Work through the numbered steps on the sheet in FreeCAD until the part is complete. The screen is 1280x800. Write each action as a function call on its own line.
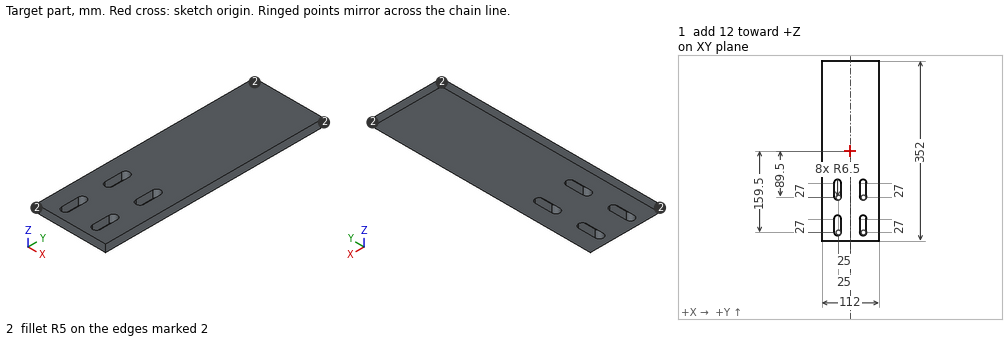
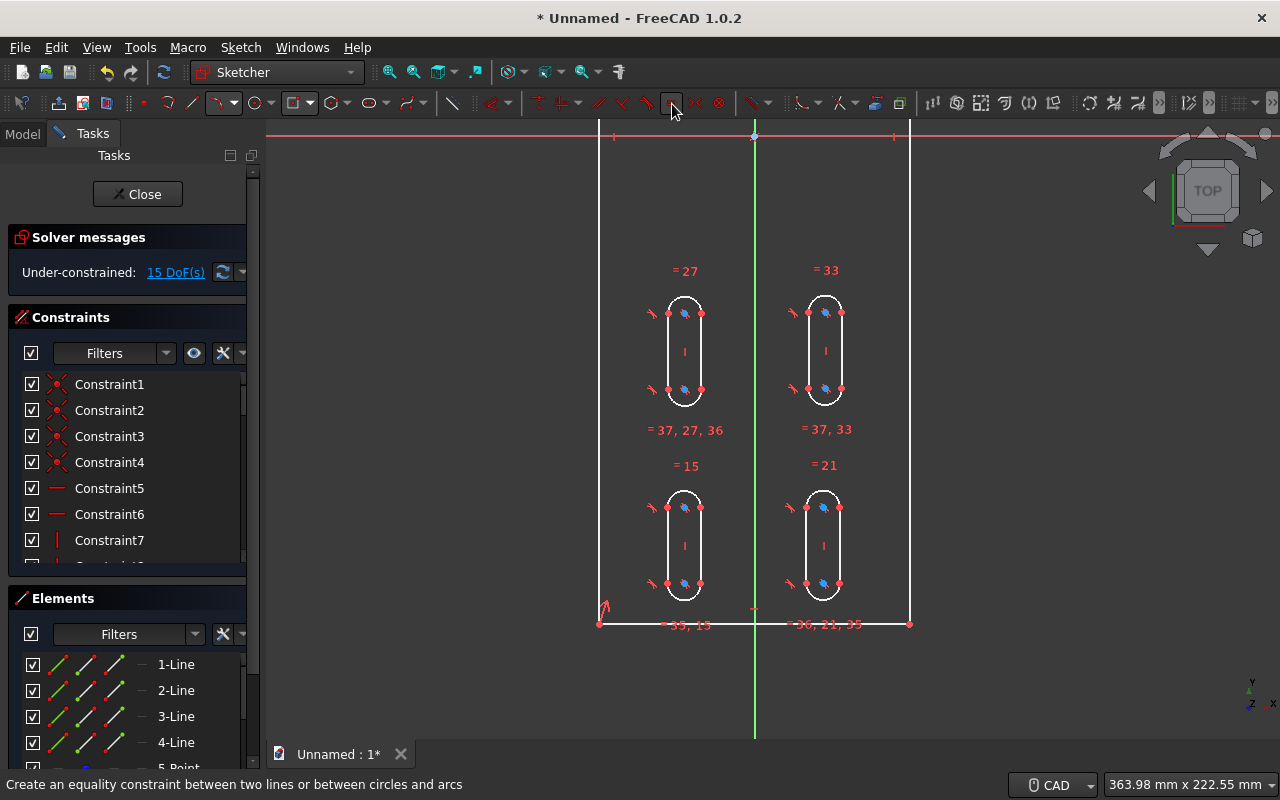
click(684, 584)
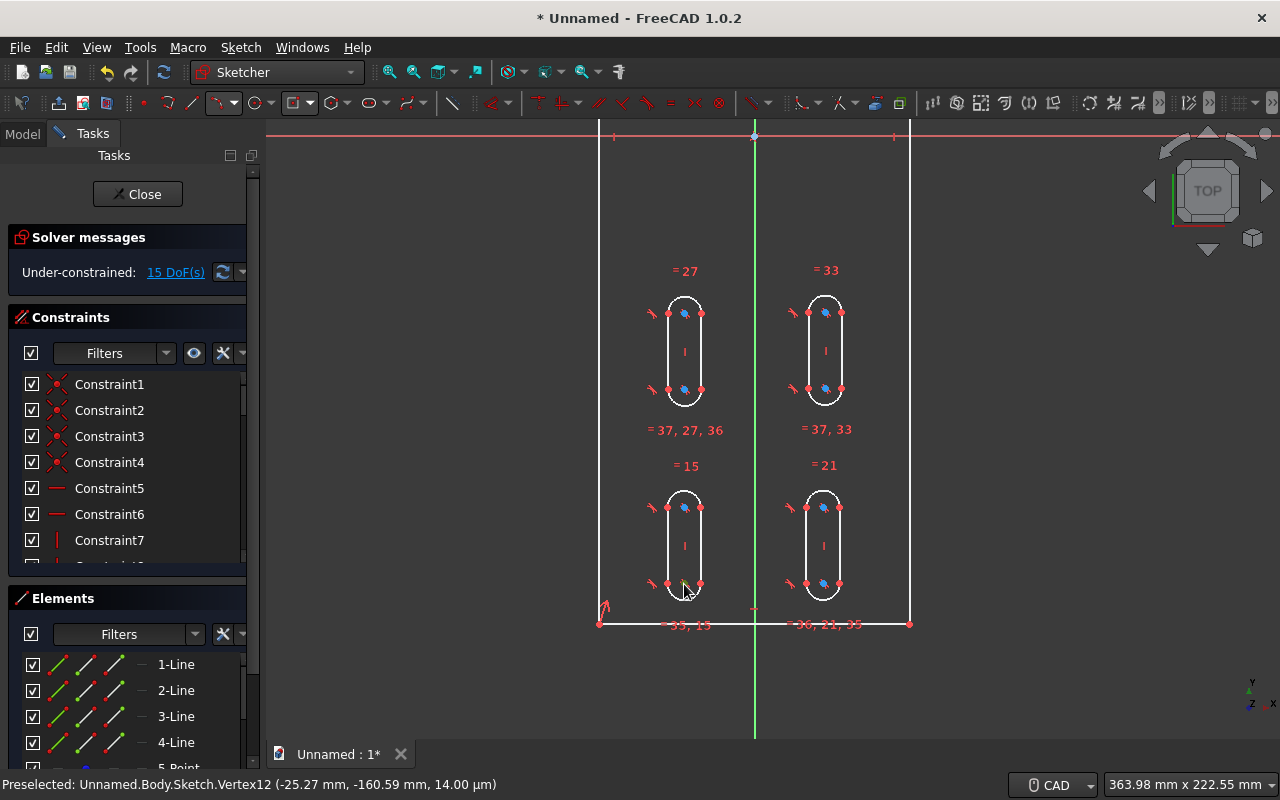
click(823, 583)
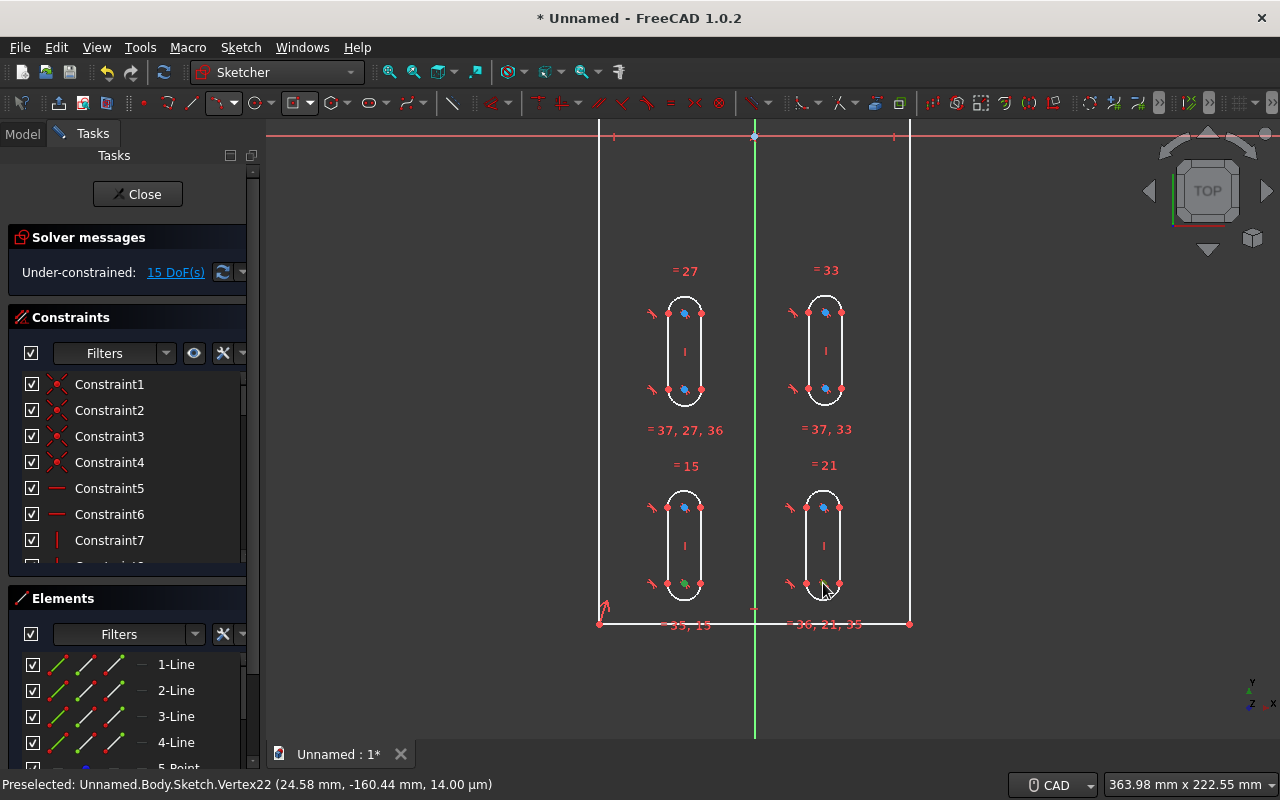
click(755, 671)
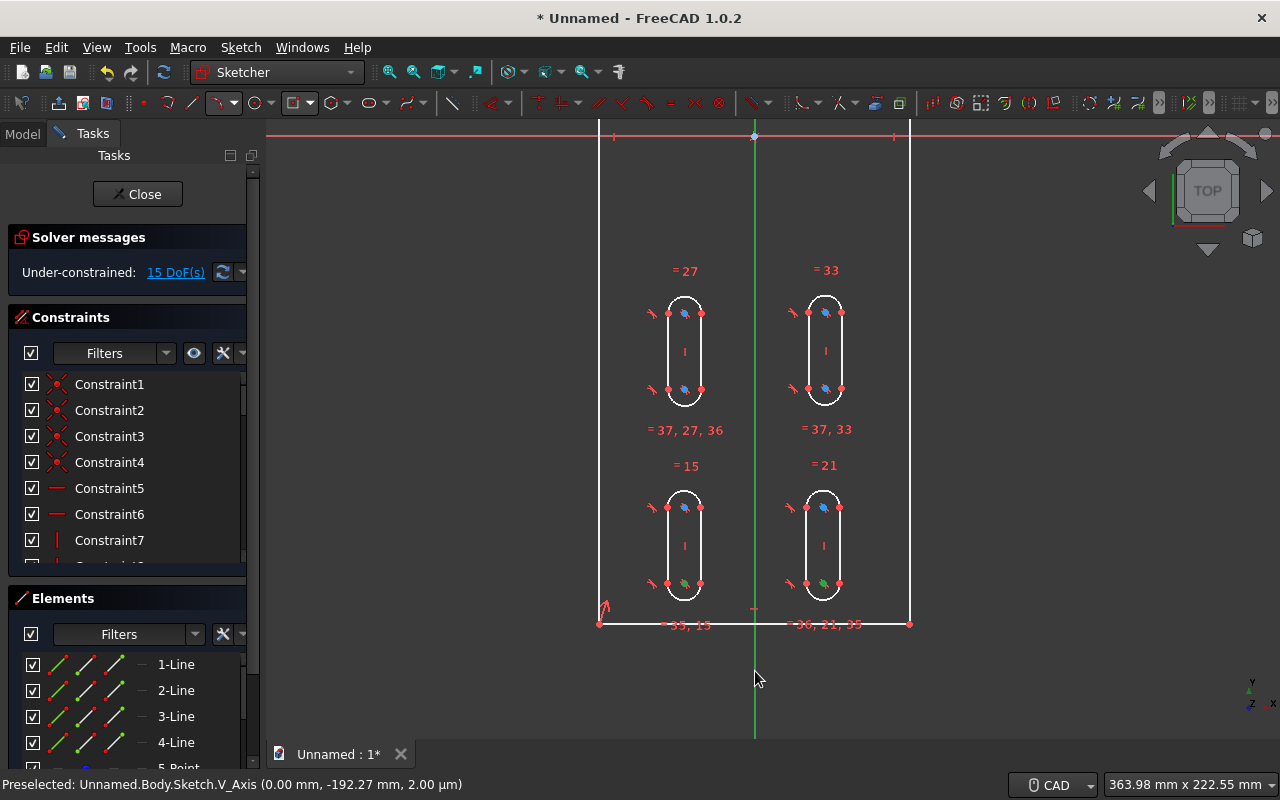
click(696, 104)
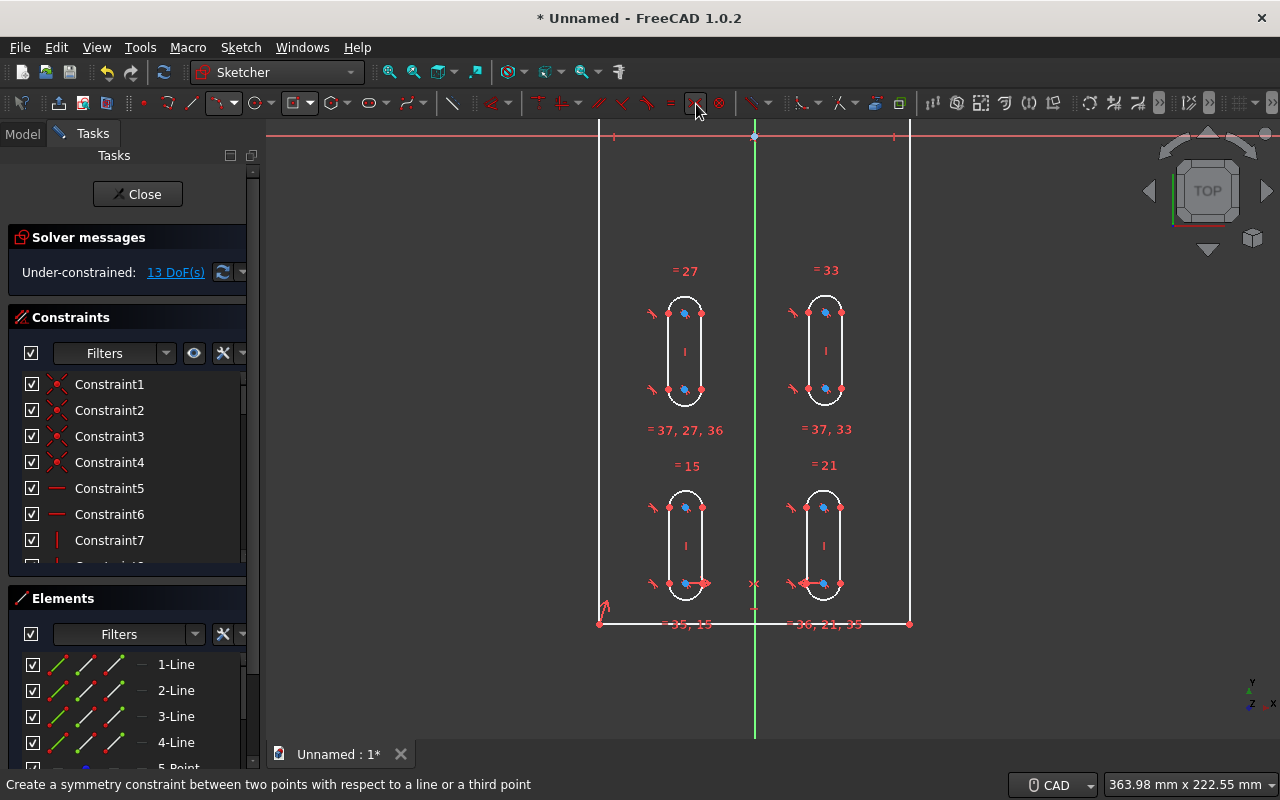
click(685, 389)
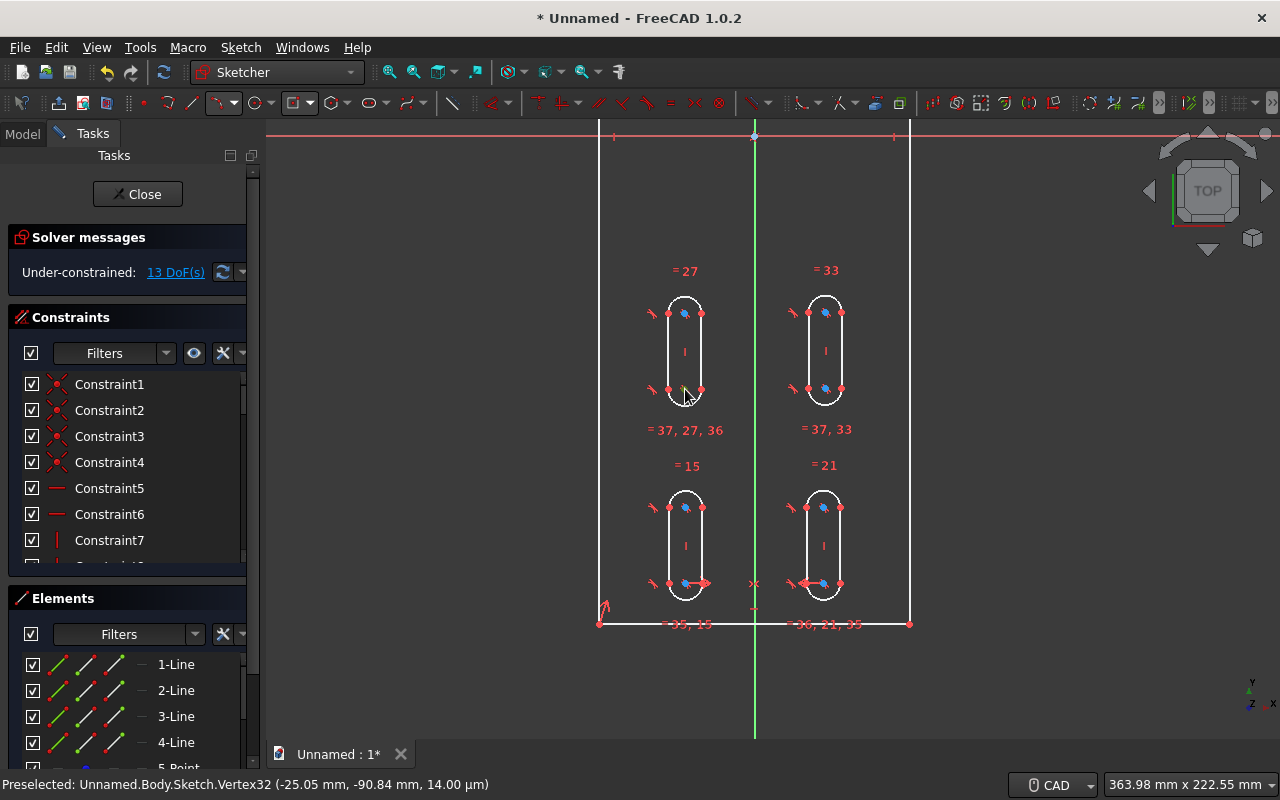
click(825, 388)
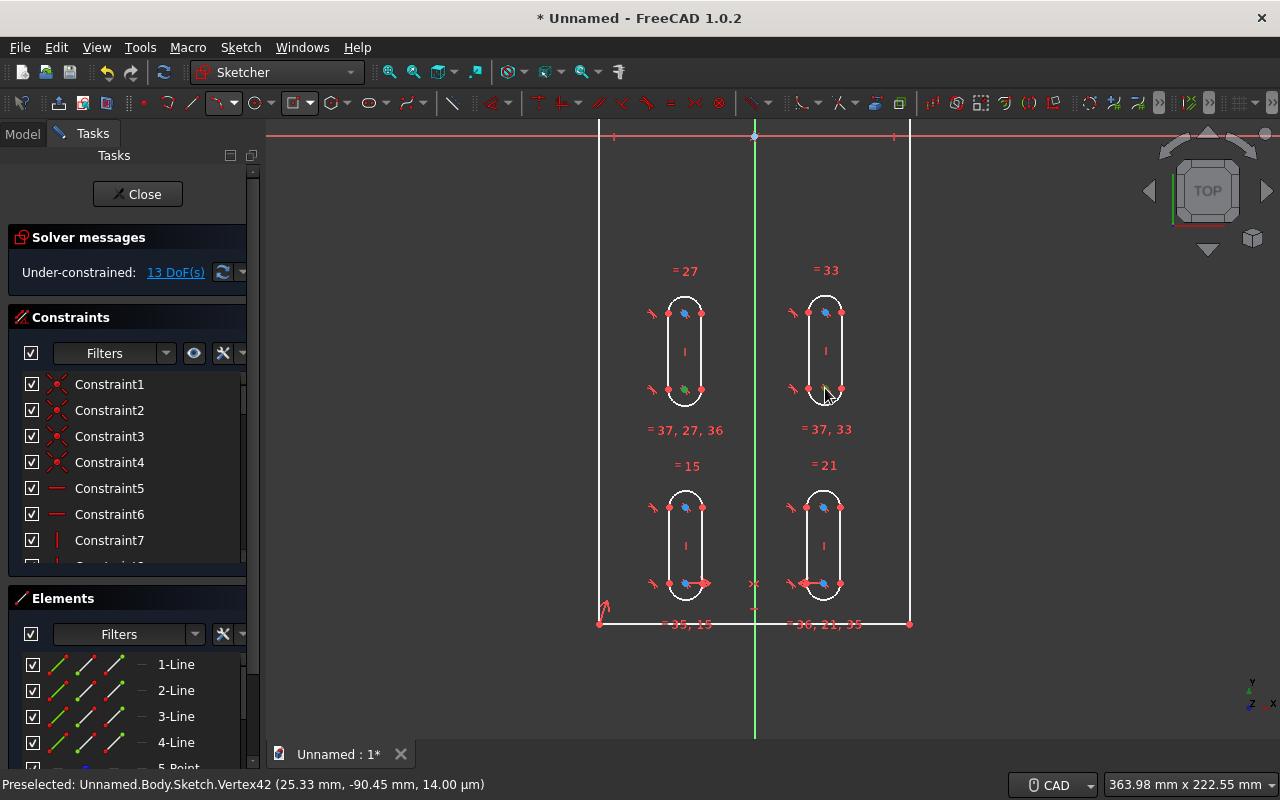
click(755, 671)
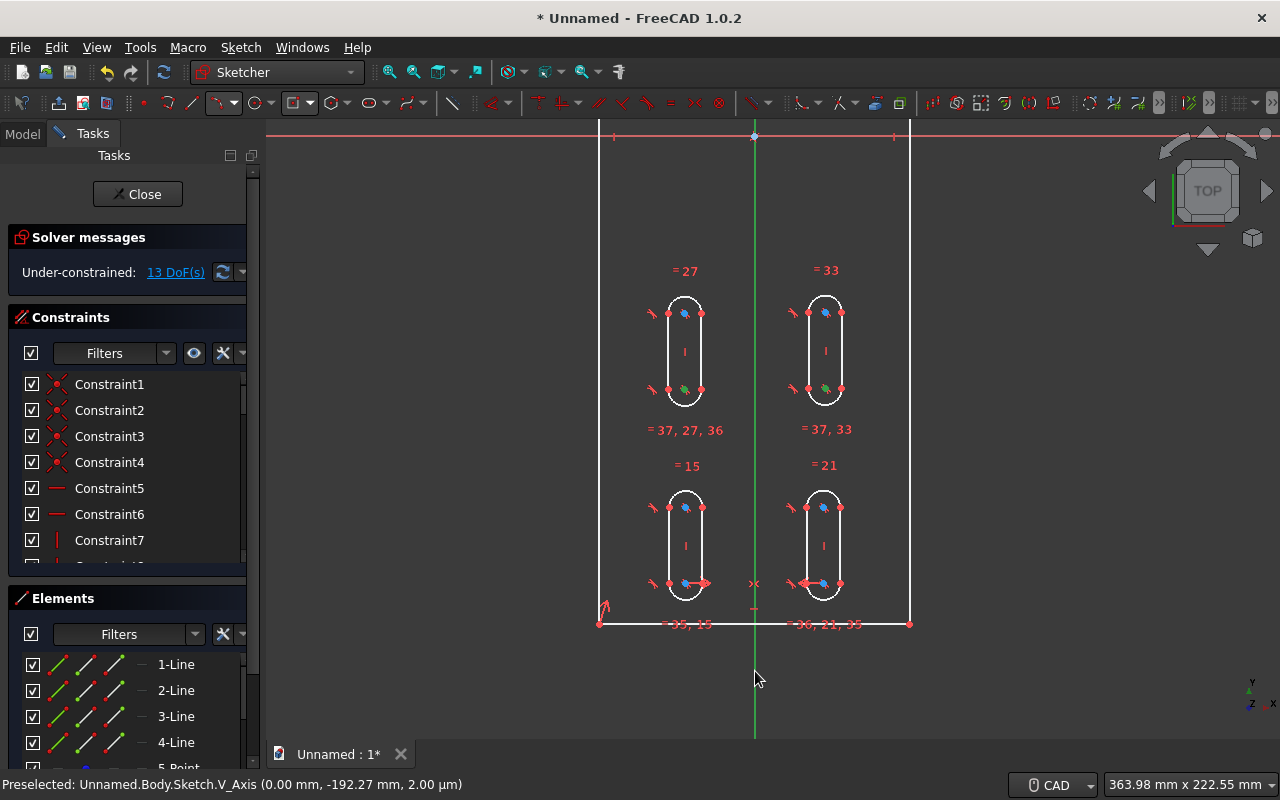
click(696, 104)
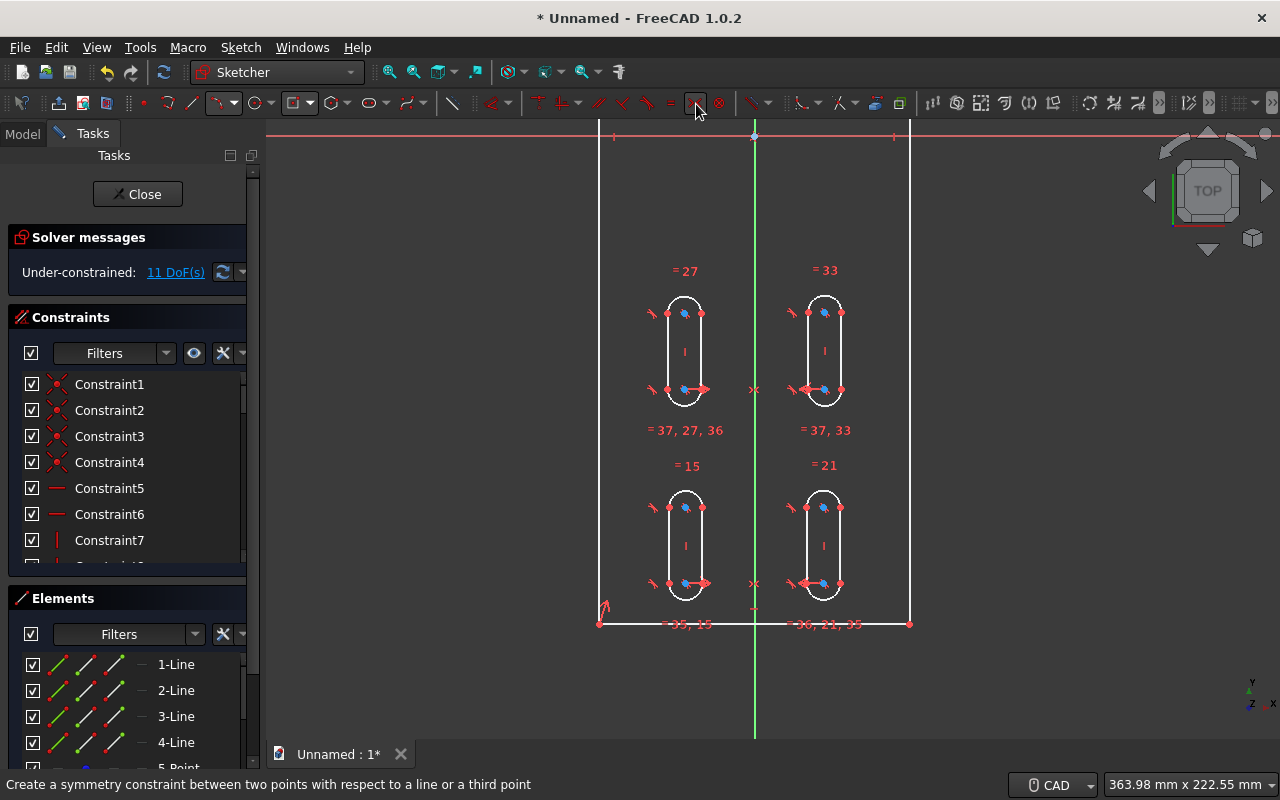
click(492, 104)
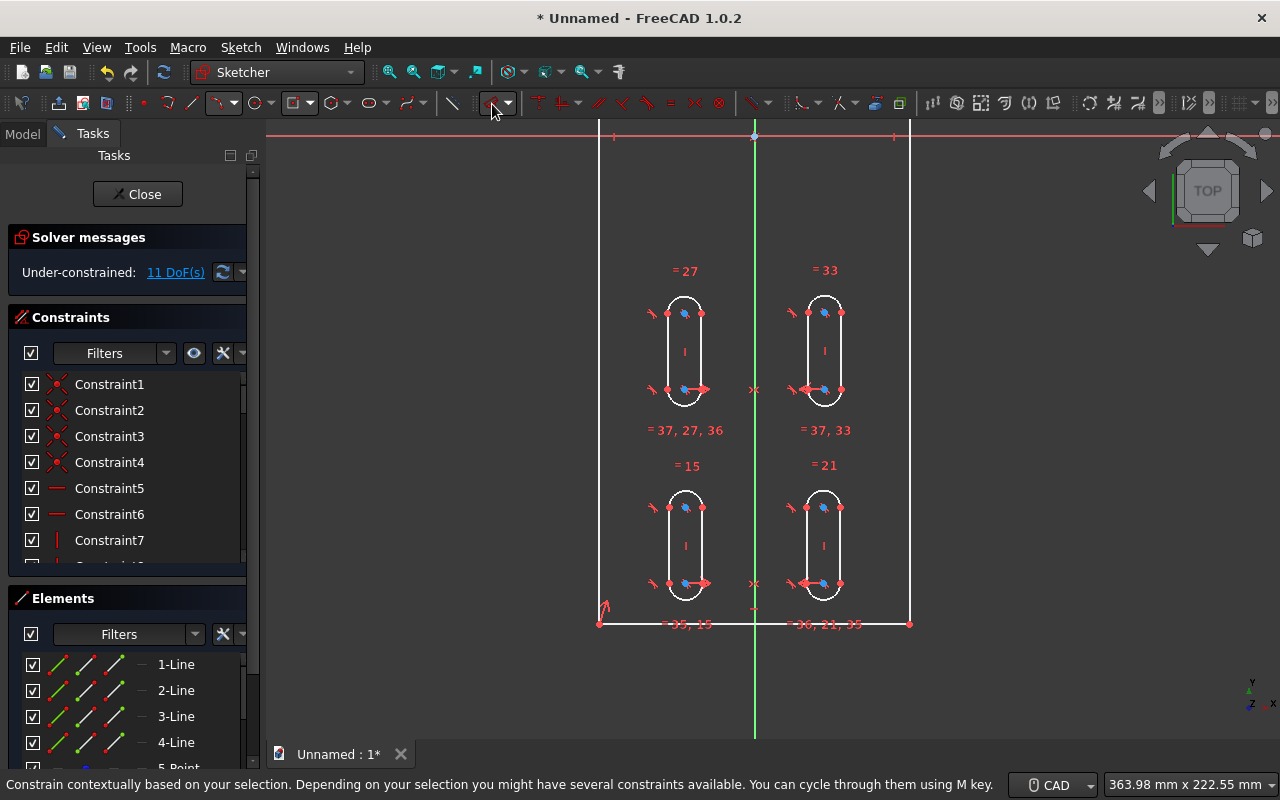
scroll(676, 597, up, 4)